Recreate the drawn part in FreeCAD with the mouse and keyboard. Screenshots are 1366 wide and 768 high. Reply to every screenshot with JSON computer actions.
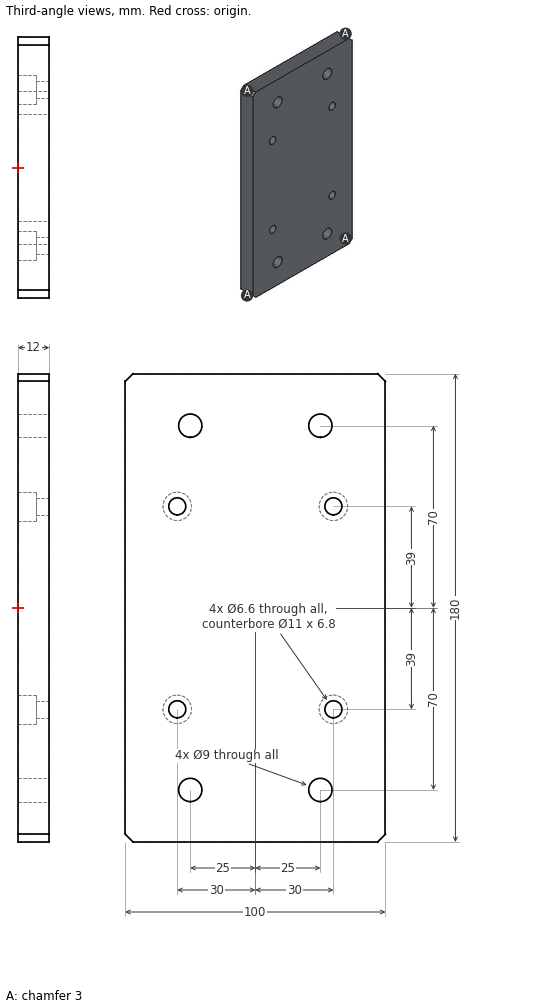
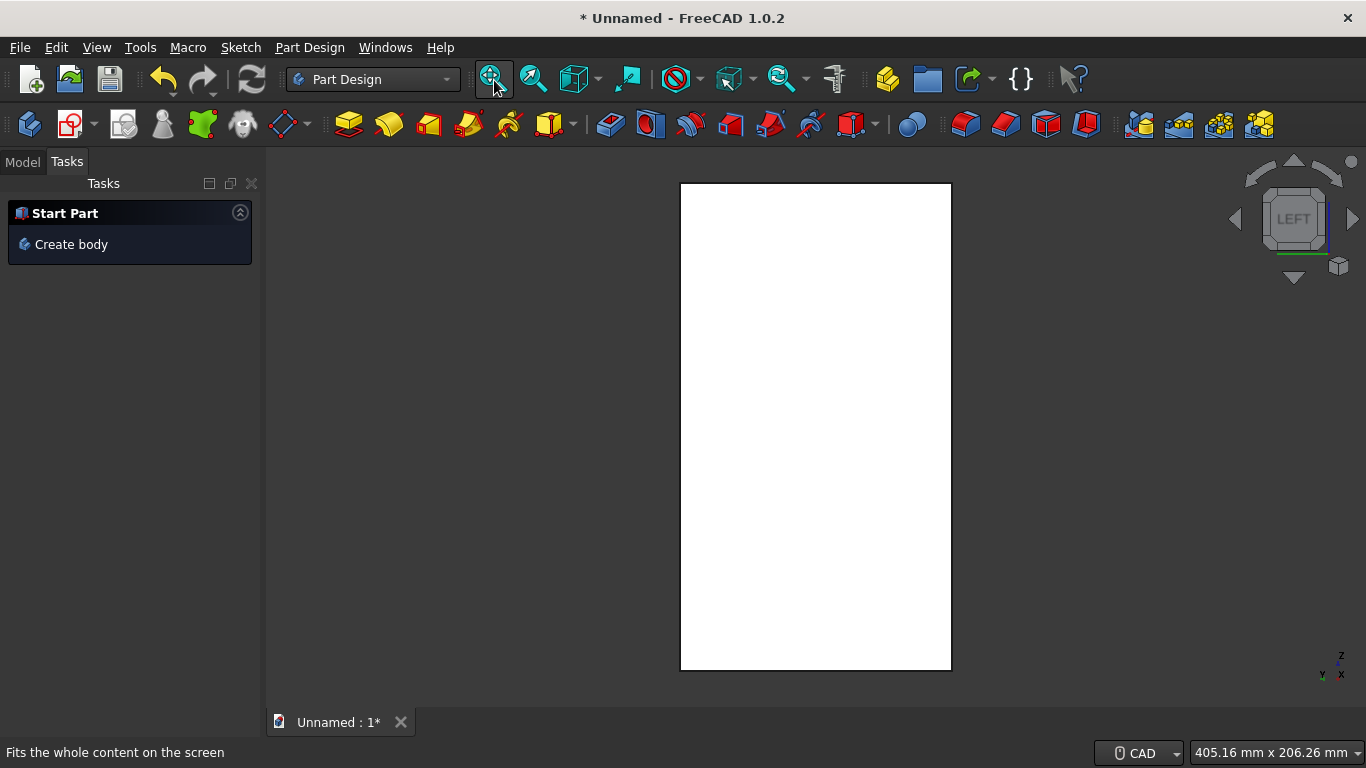
{"action": "left_click", "coordinate": [816, 496]}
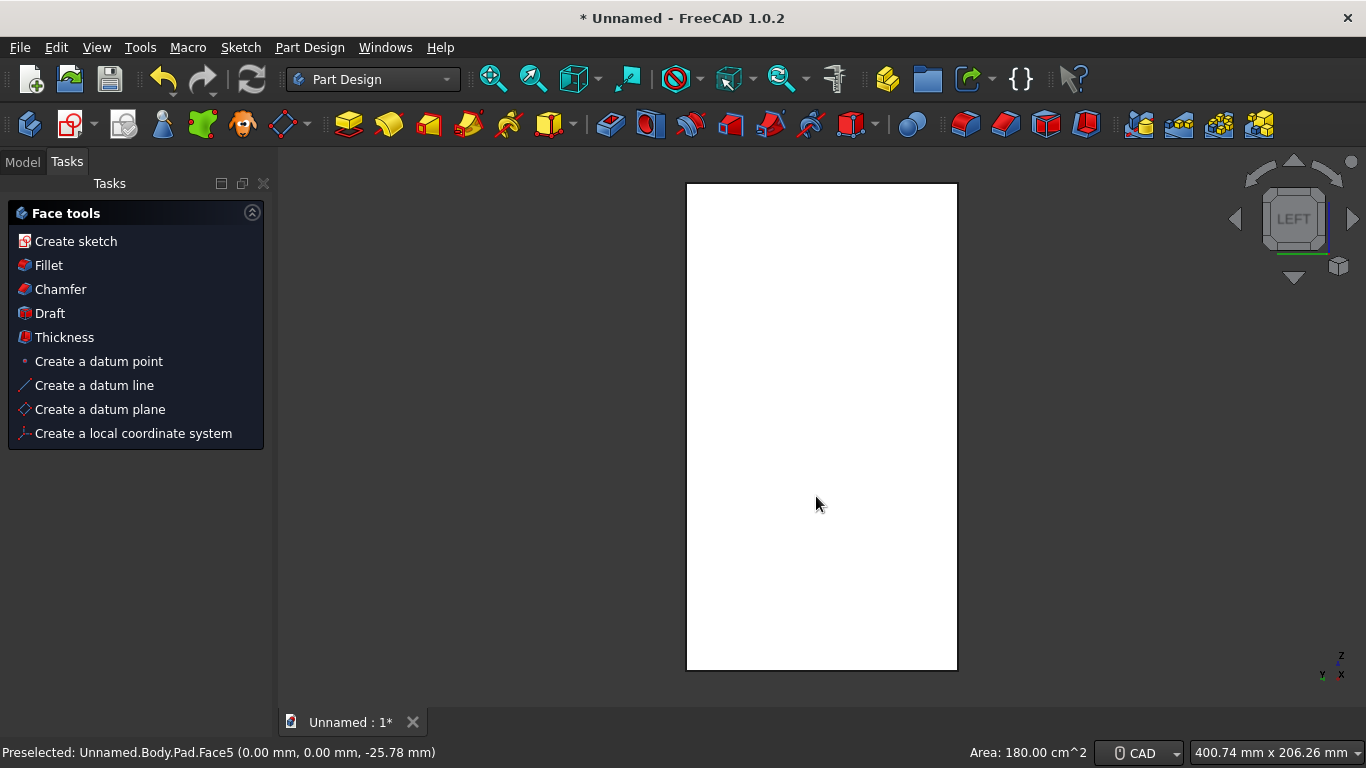
{"action": "left_click", "coordinate": [70, 124]}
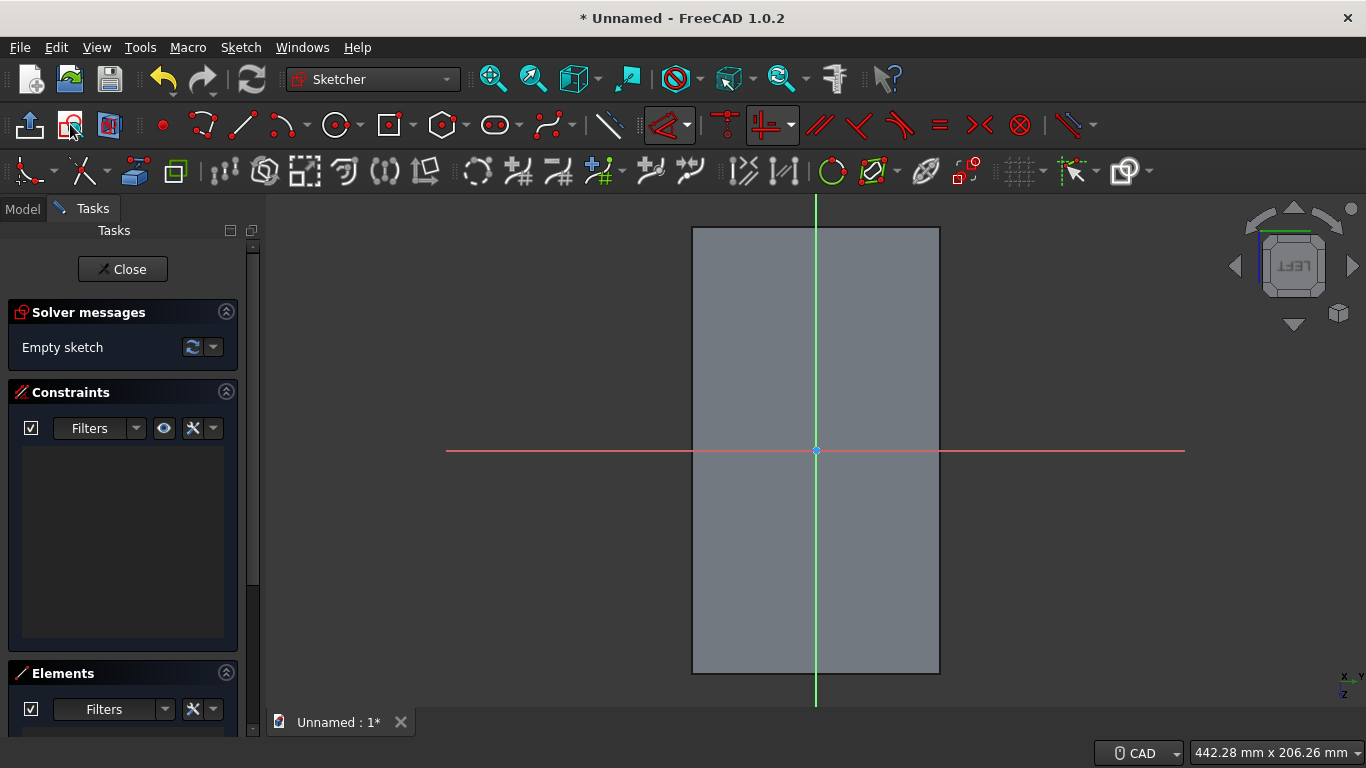
{"action": "scroll", "coordinate": [955, 451], "scroll_direction": "up", "scroll_amount": 2}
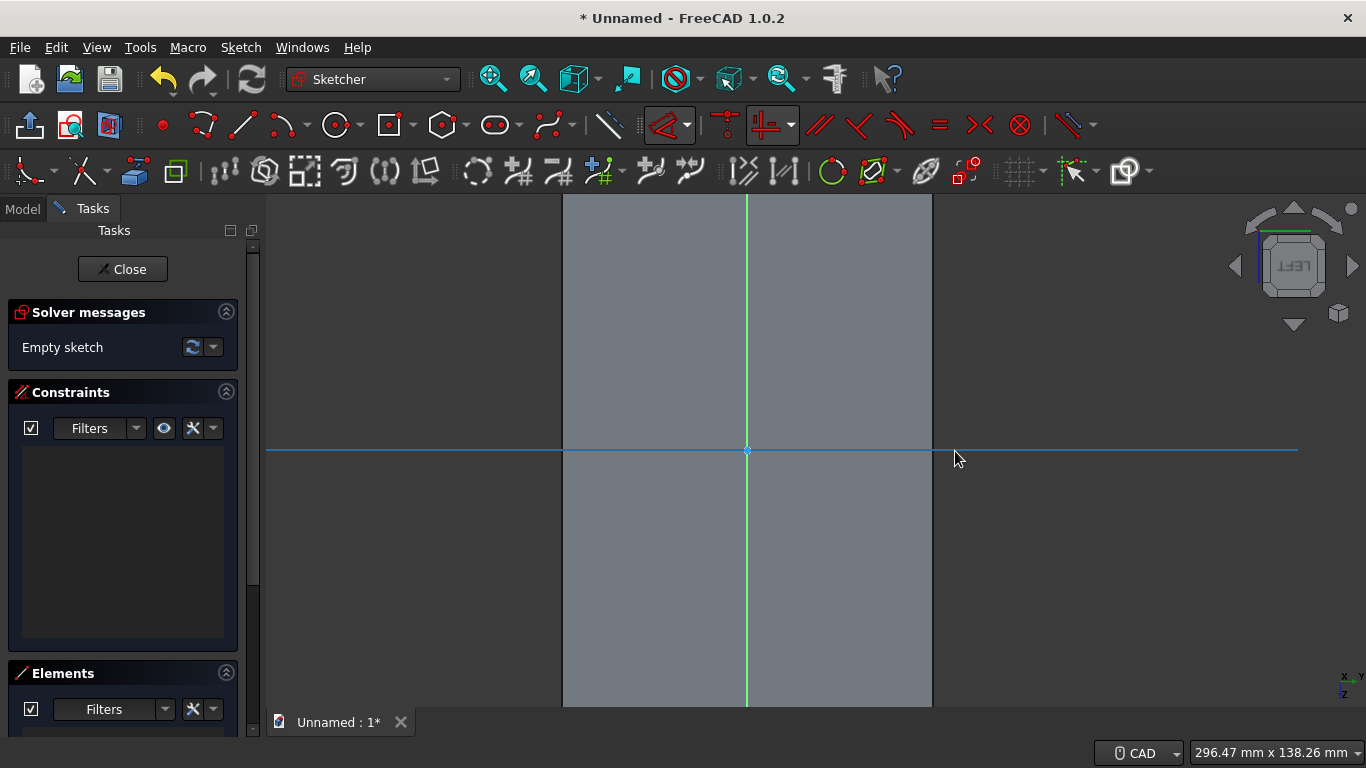
{"action": "left_click", "coordinate": [336, 126]}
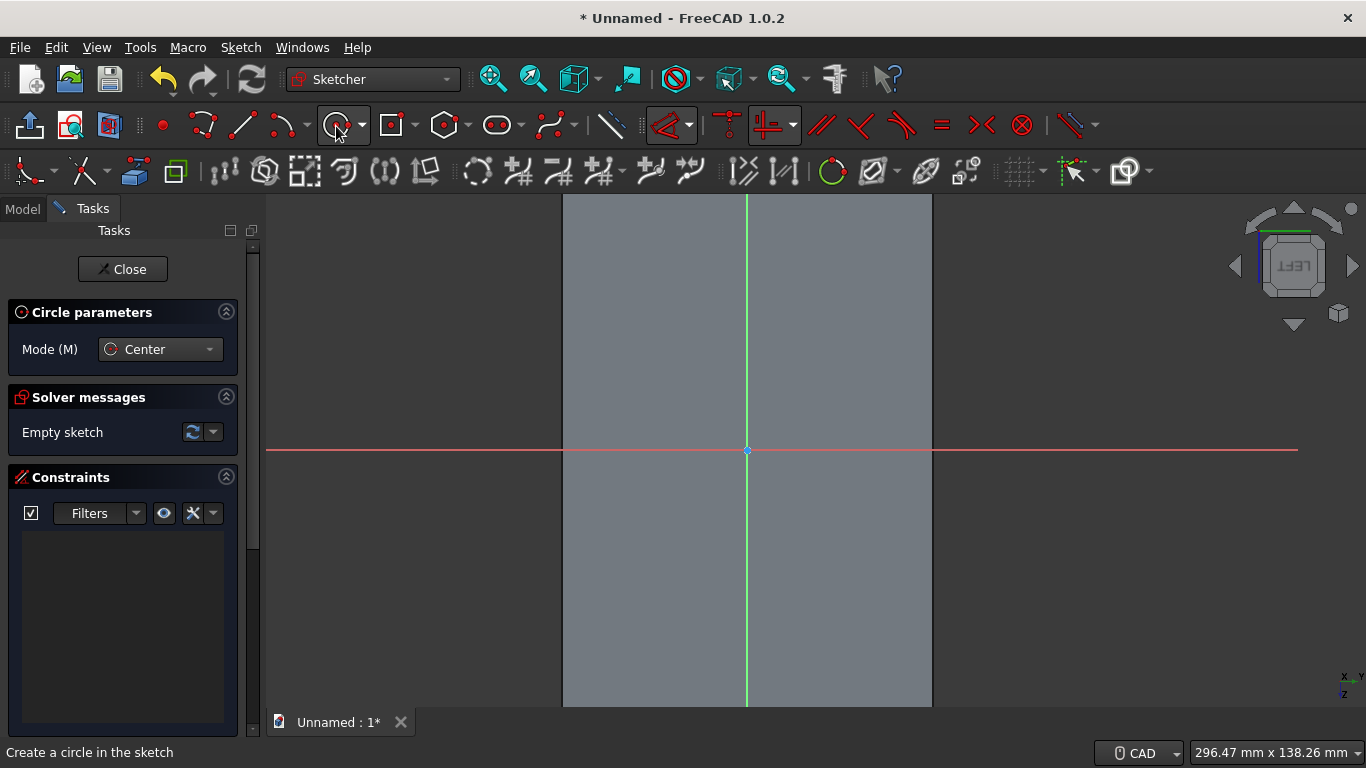
{"action": "scroll", "coordinate": [859, 305], "scroll_direction": "up", "scroll_amount": 4}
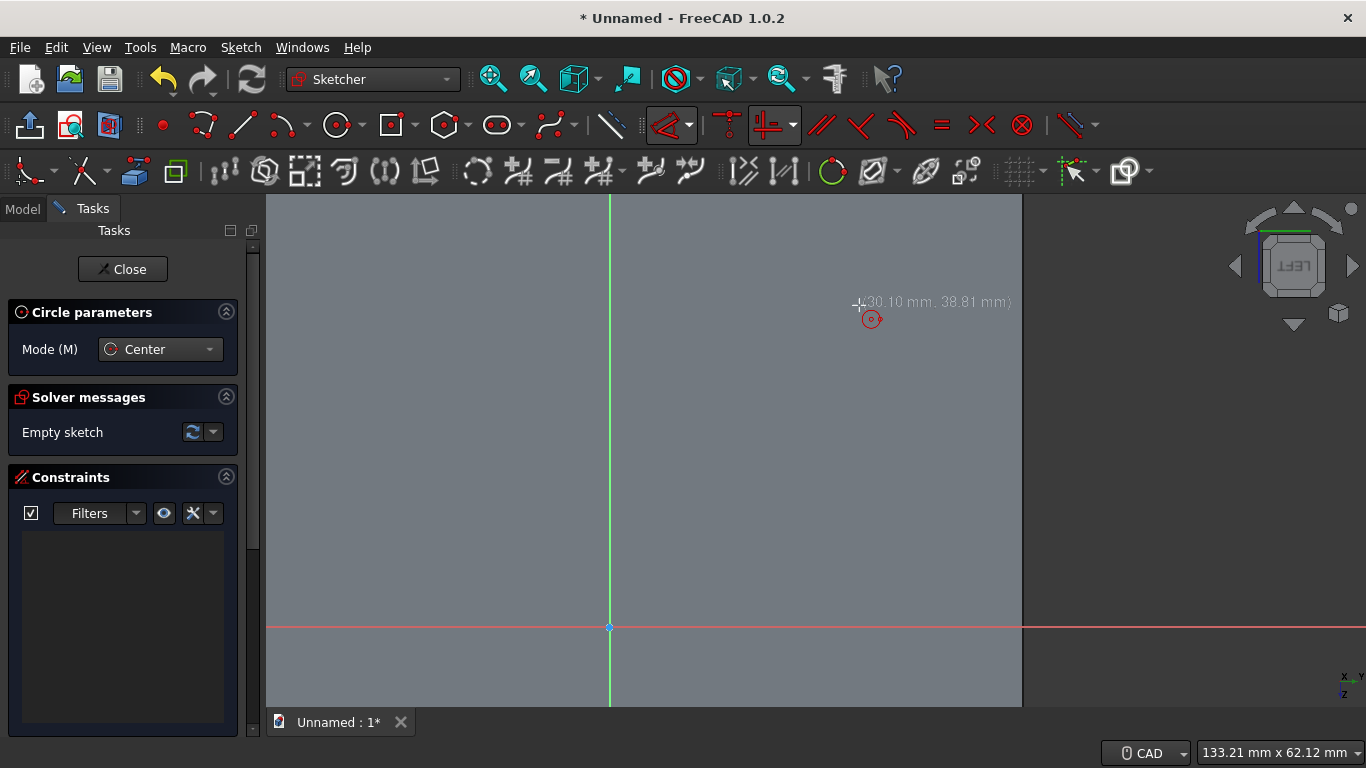
{"action": "left_click", "coordinate": [858, 305]}
{"action": "left_click", "coordinate": [877, 286]}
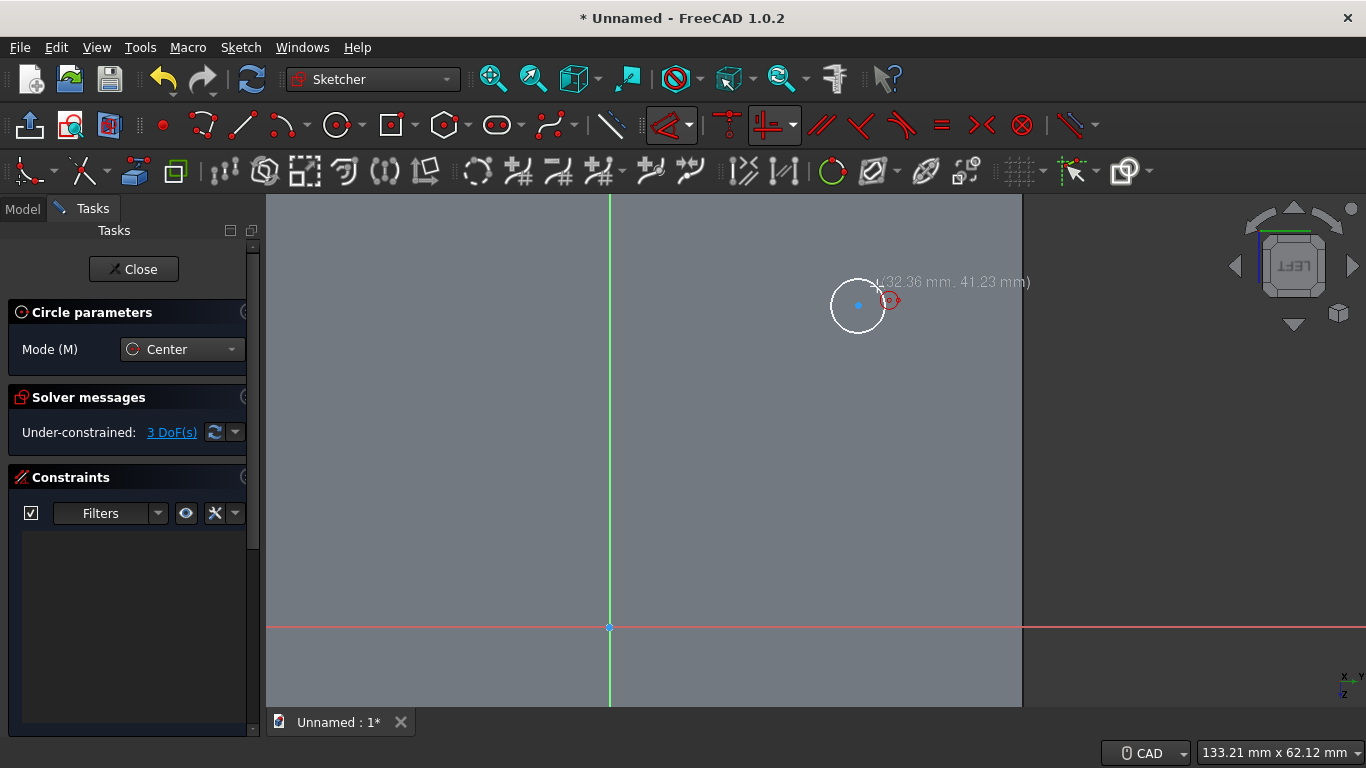
{"action": "left_click", "coordinate": [362, 305]}
{"action": "left_click", "coordinate": [381, 286]}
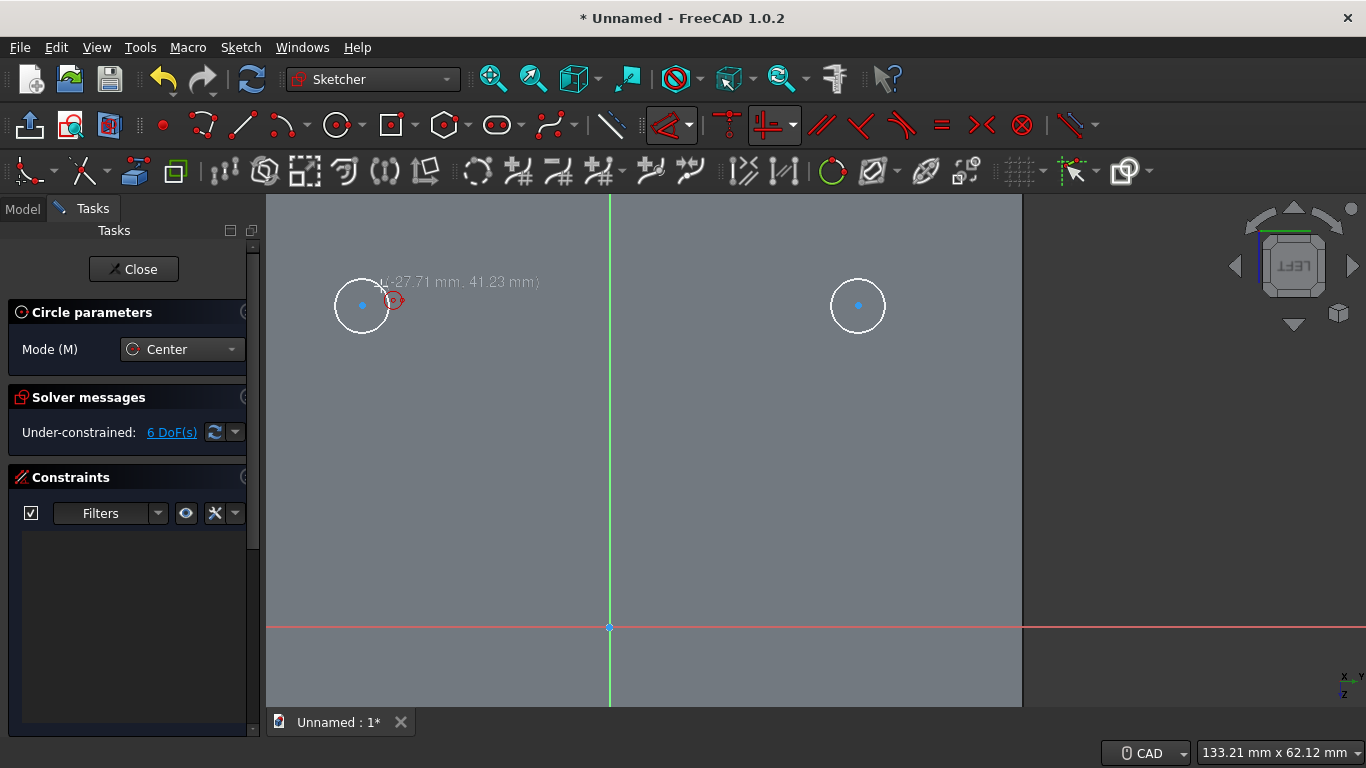
{"action": "scroll", "coordinate": [860, 306], "scroll_direction": "down", "scroll_amount": 4}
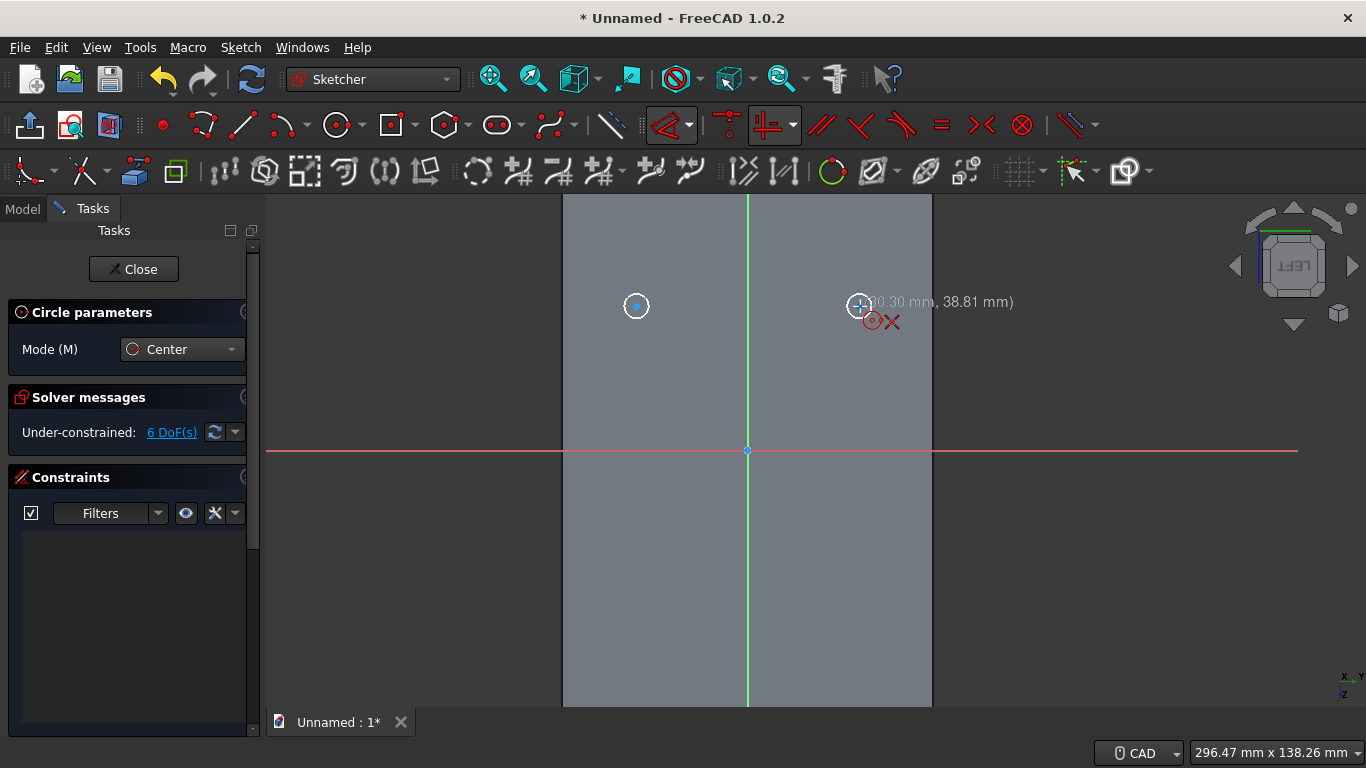
{"action": "scroll", "coordinate": [859, 595], "scroll_direction": "up", "scroll_amount": 4}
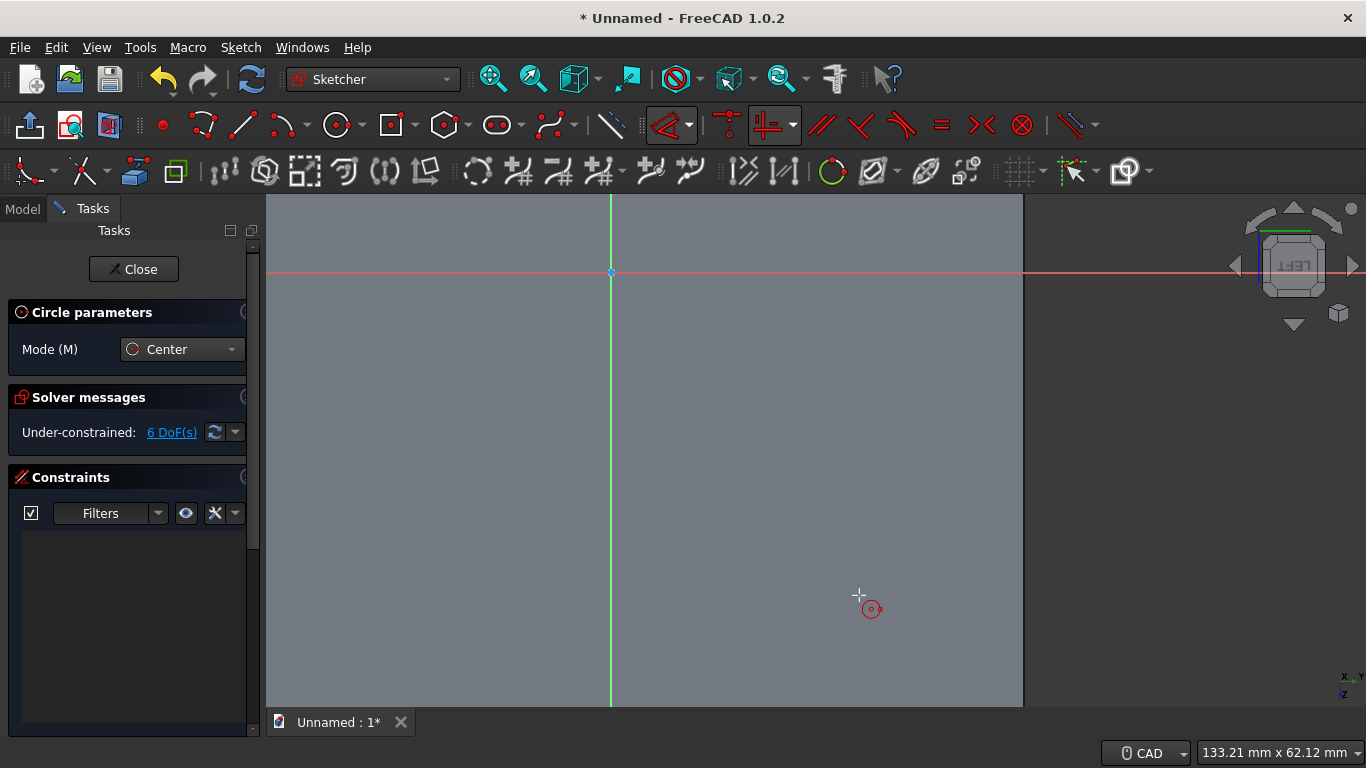
{"action": "left_click", "coordinate": [859, 595]}
{"action": "left_click", "coordinate": [878, 575]}